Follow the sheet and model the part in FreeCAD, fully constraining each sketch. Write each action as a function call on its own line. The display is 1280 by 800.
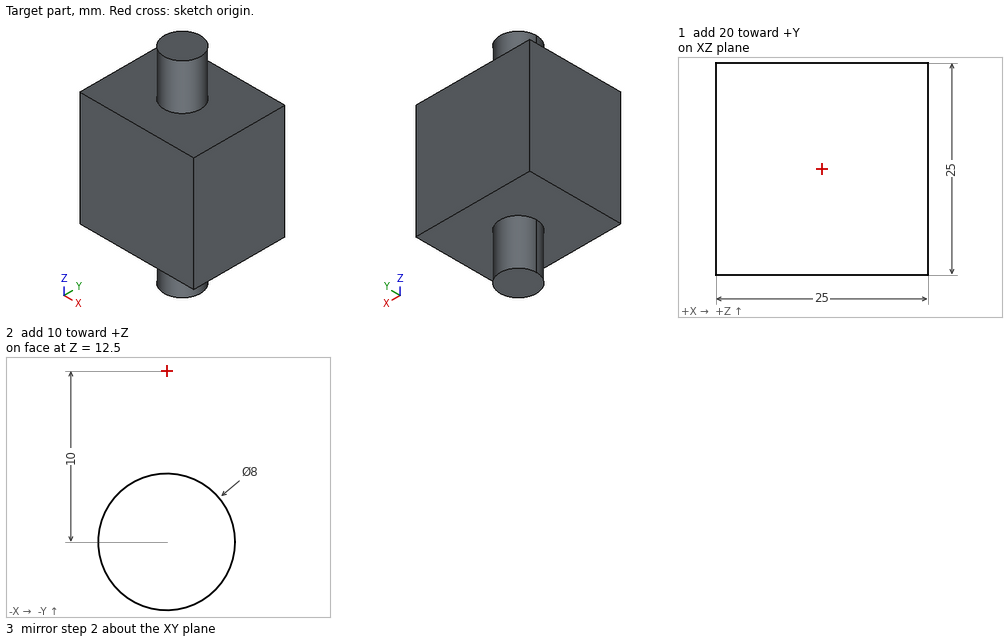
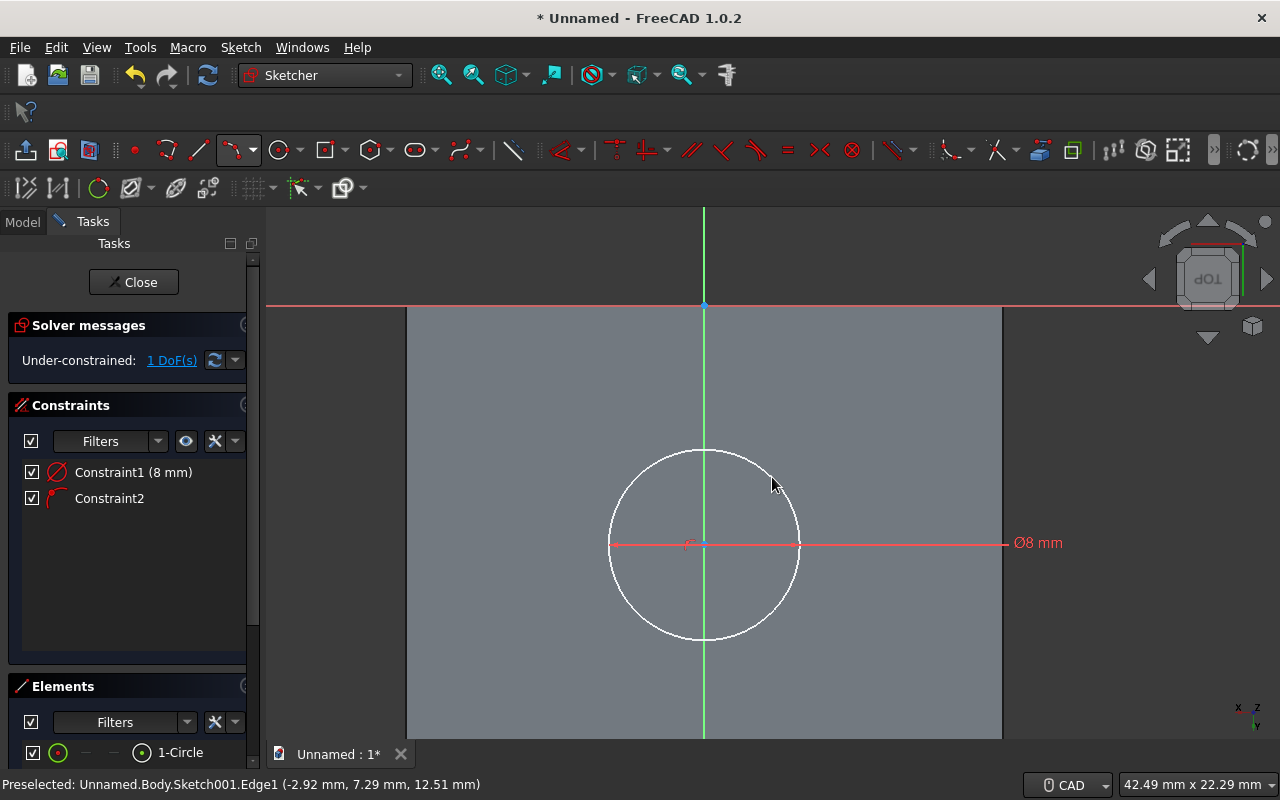
click(704, 545)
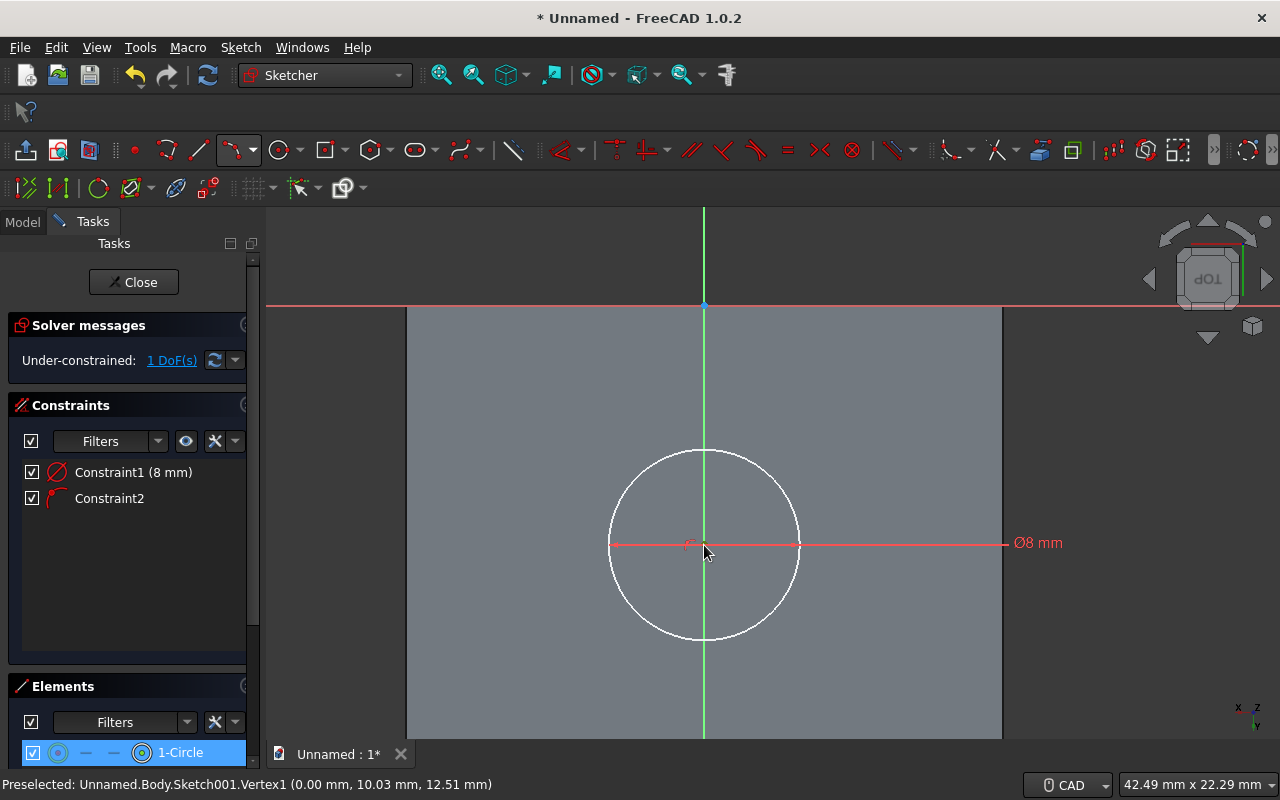
key(i)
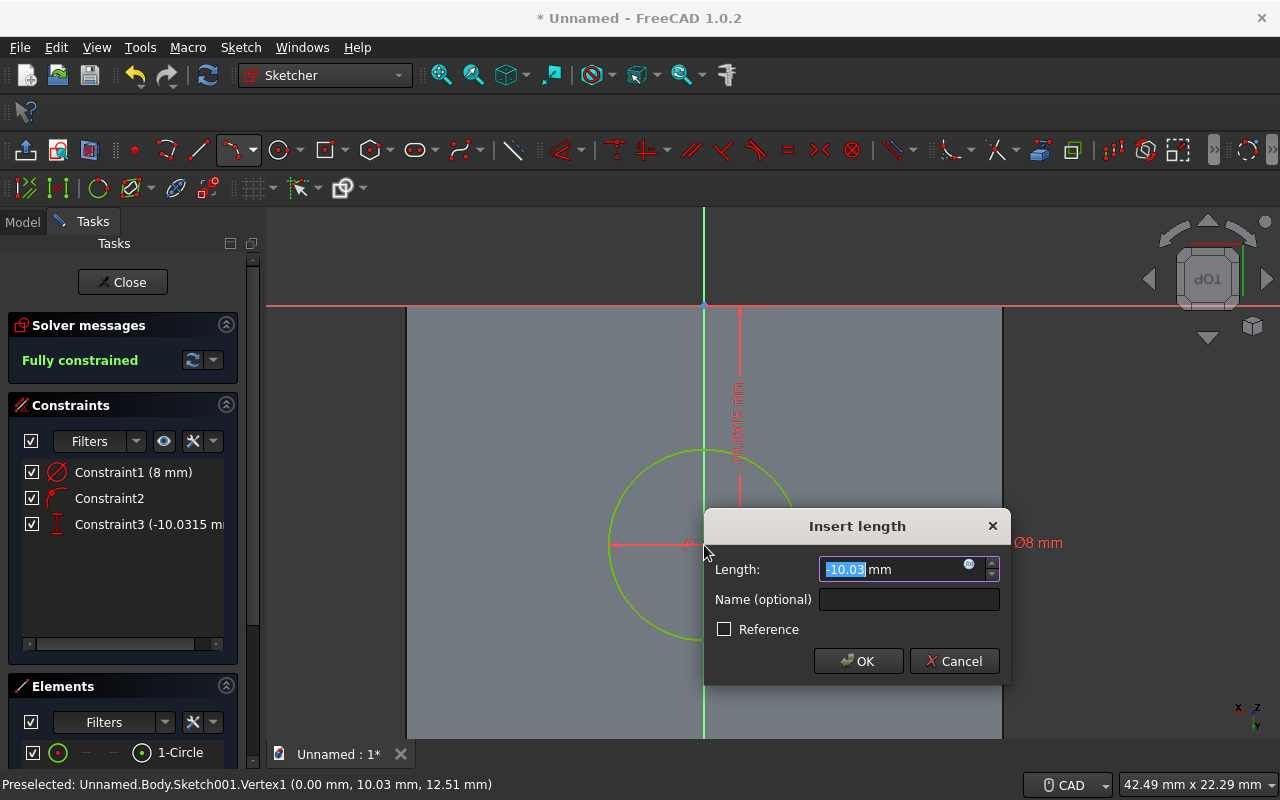
text(-10)
key(Return)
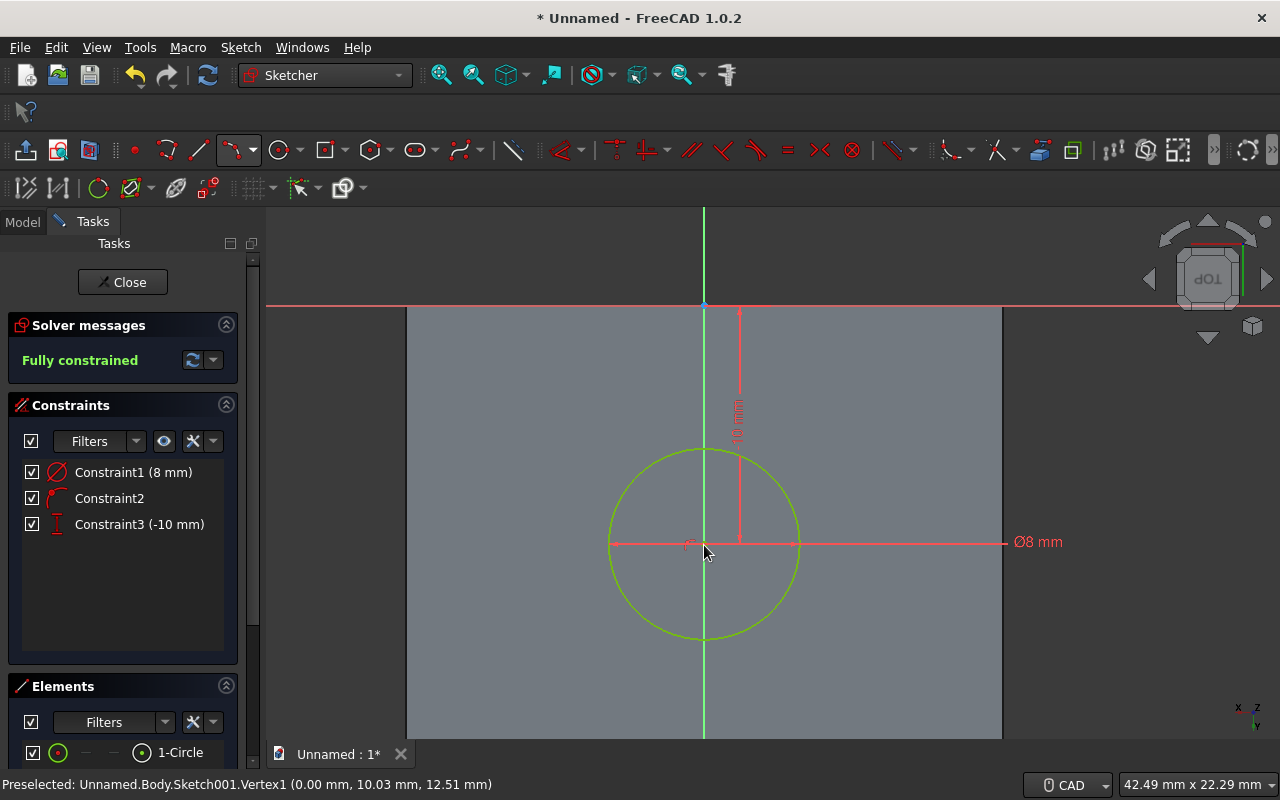
click(123, 282)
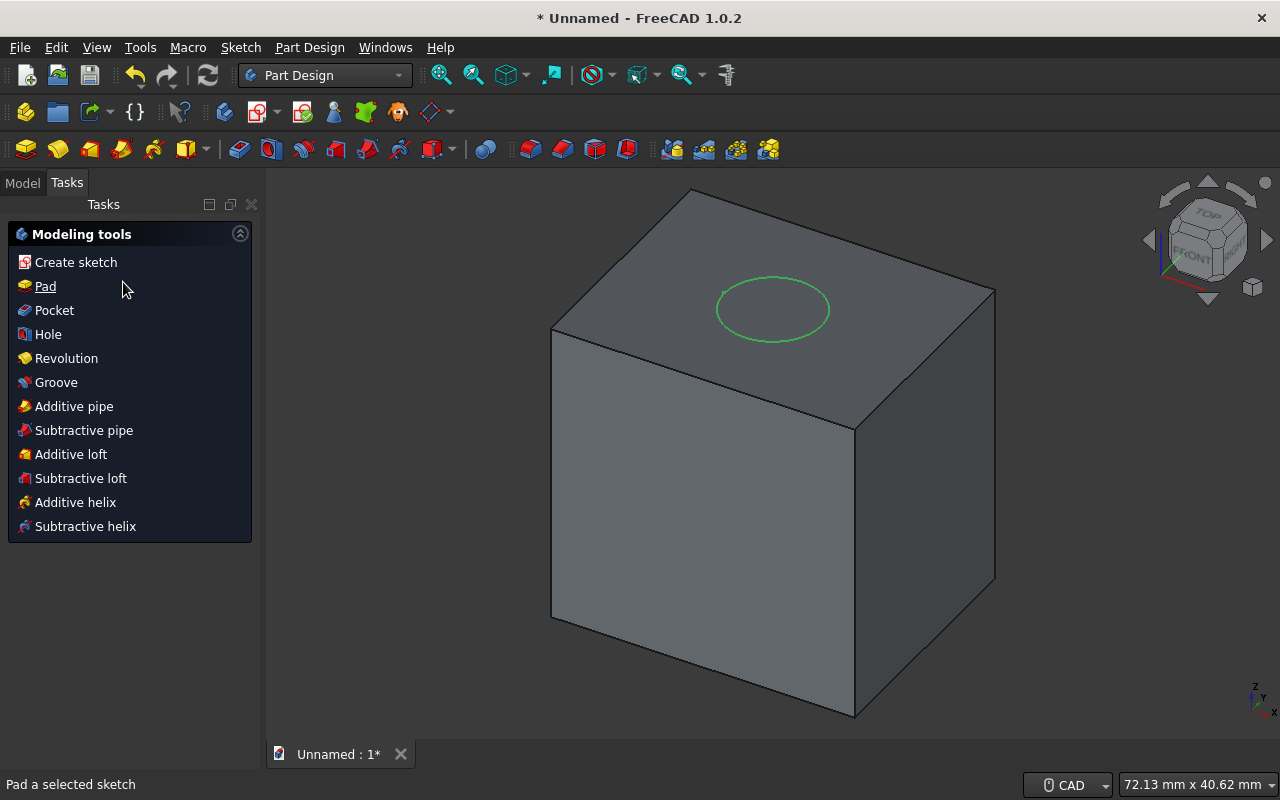
click(26, 150)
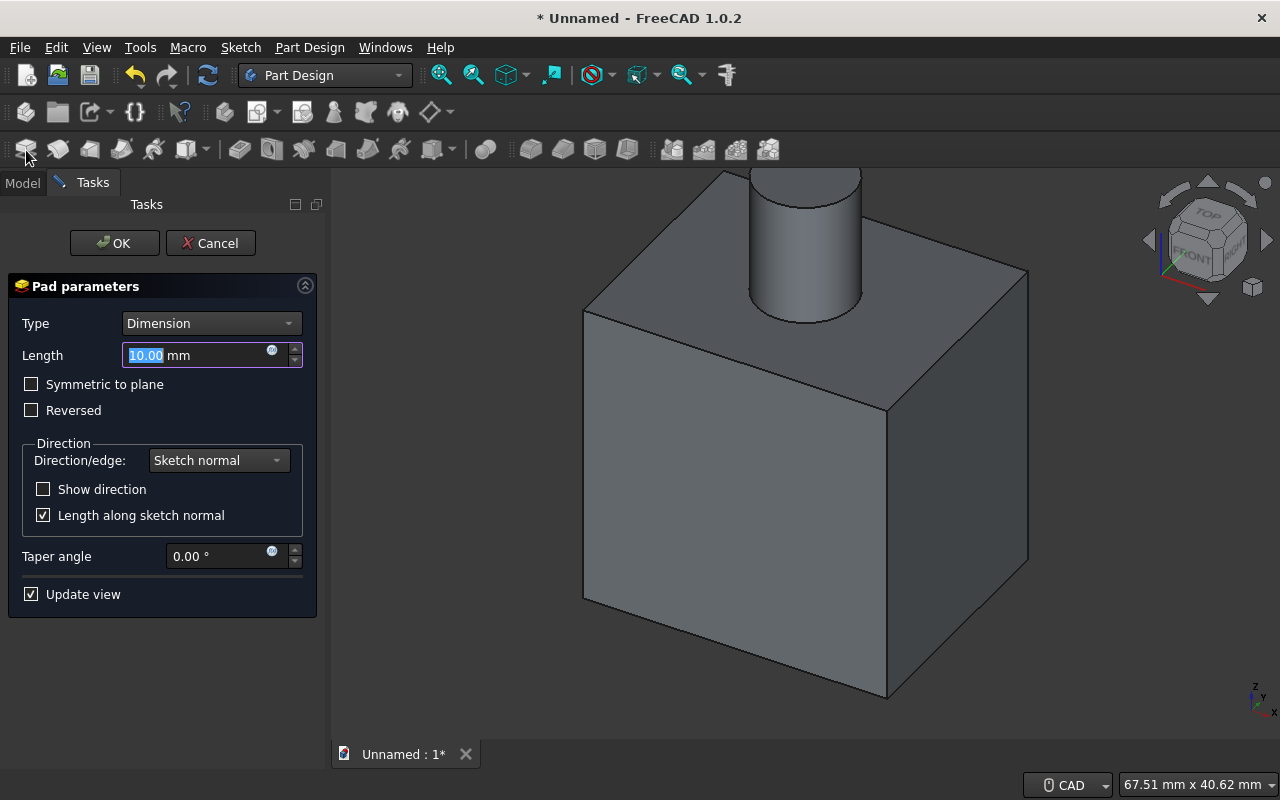
text(10)
key(Tab)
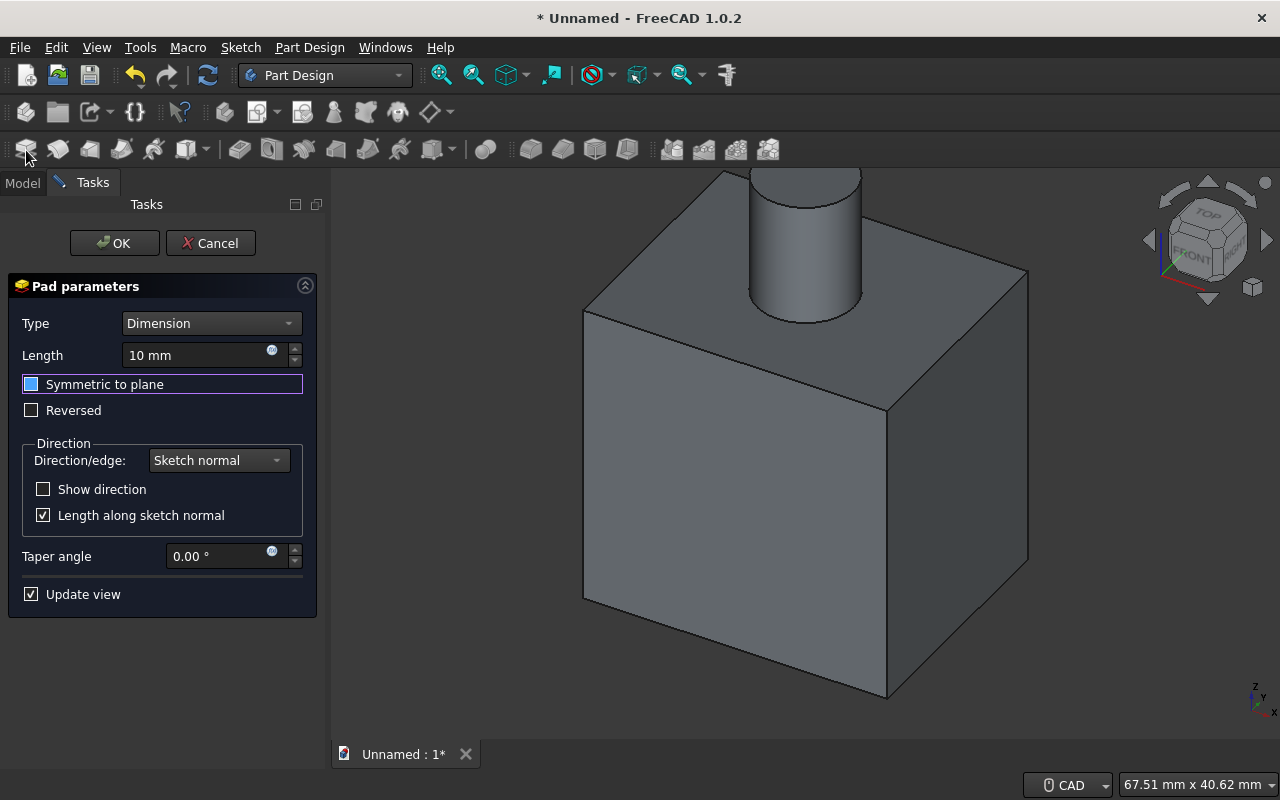
click(115, 243)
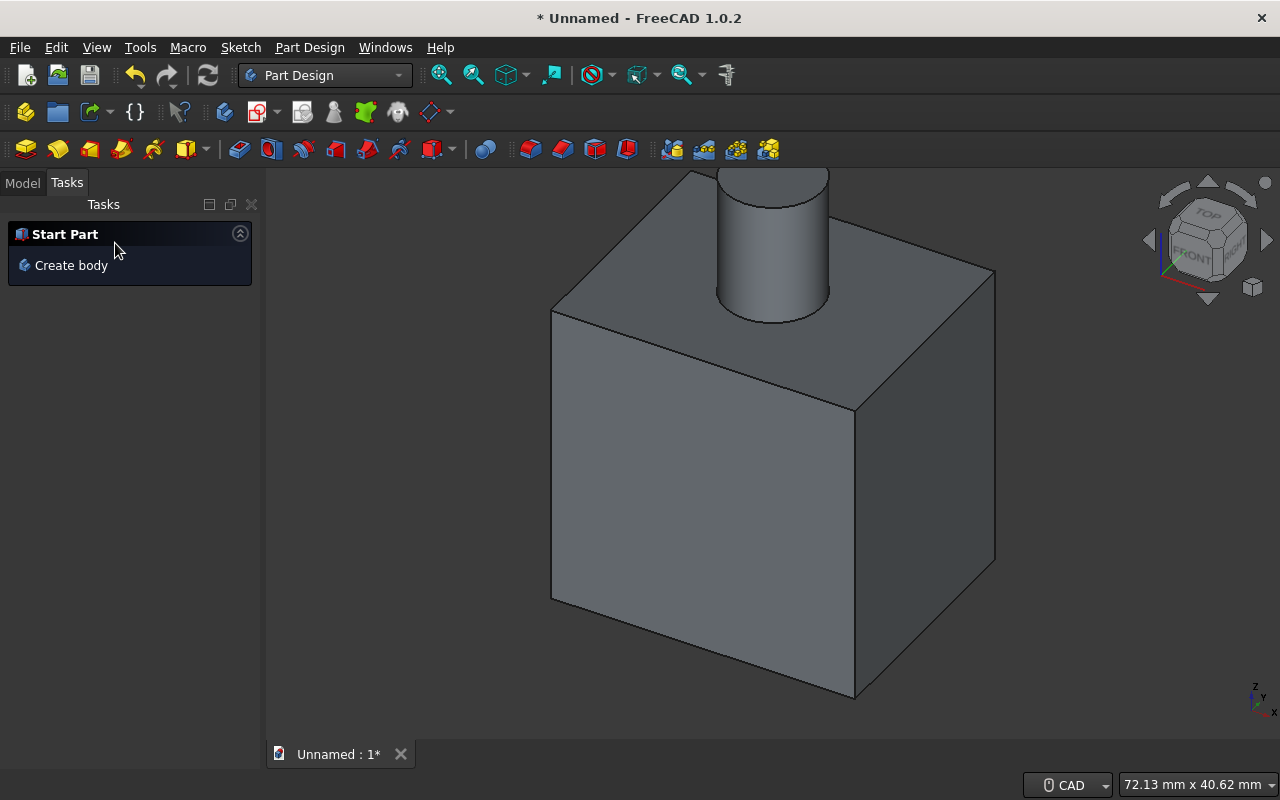
click(442, 76)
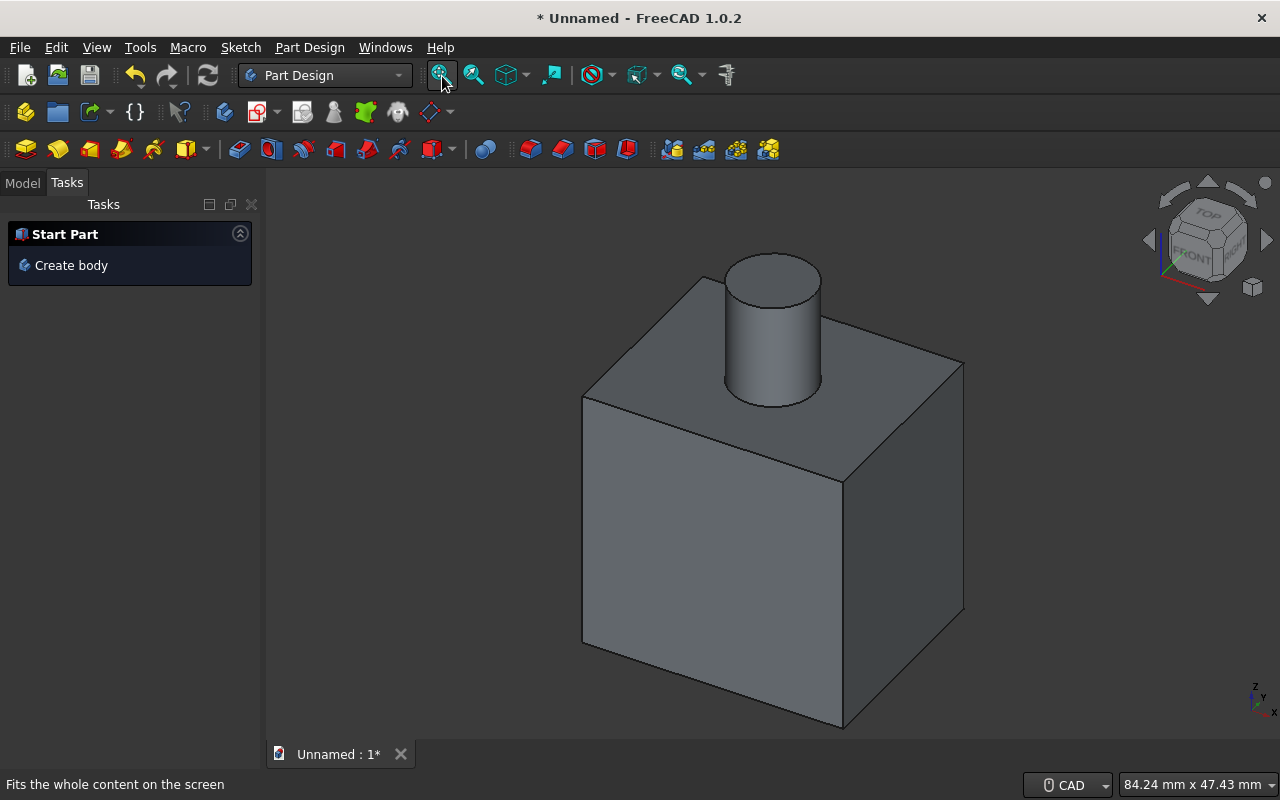
click(23, 182)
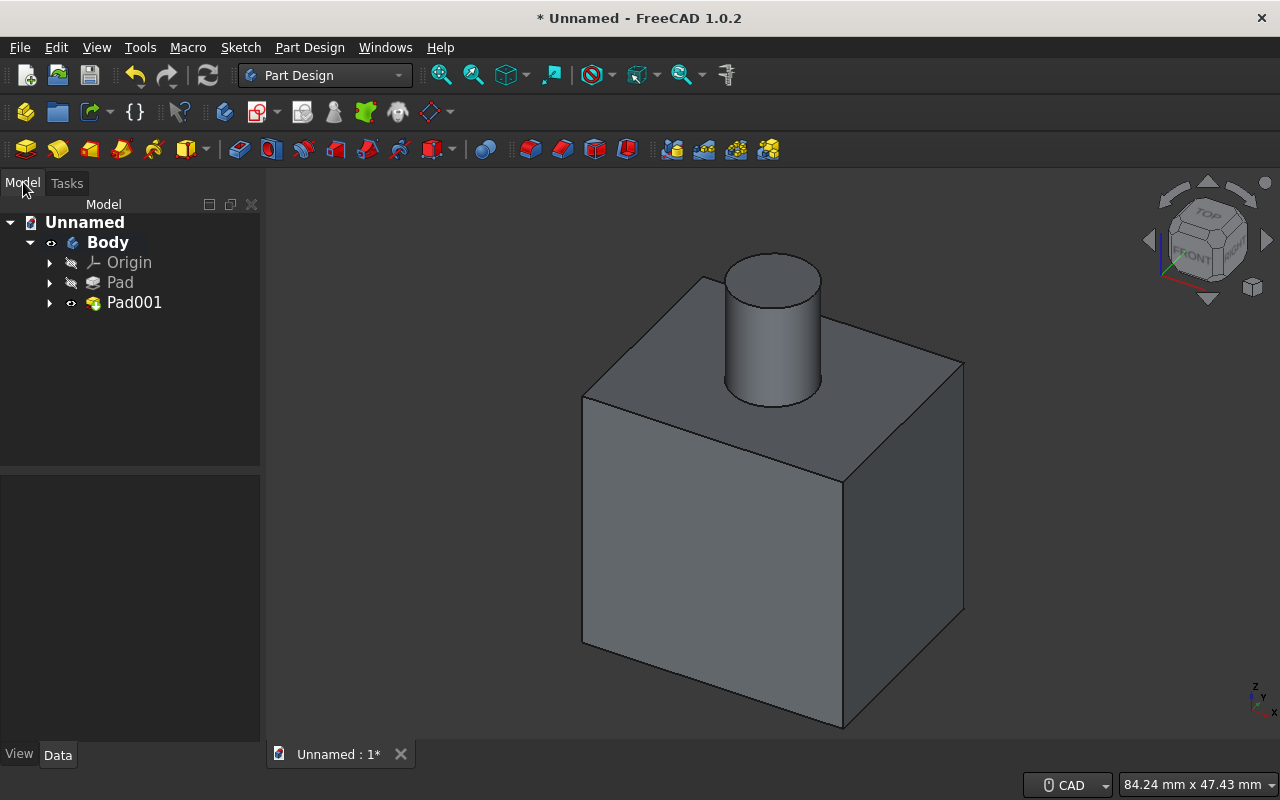
click(116, 303)